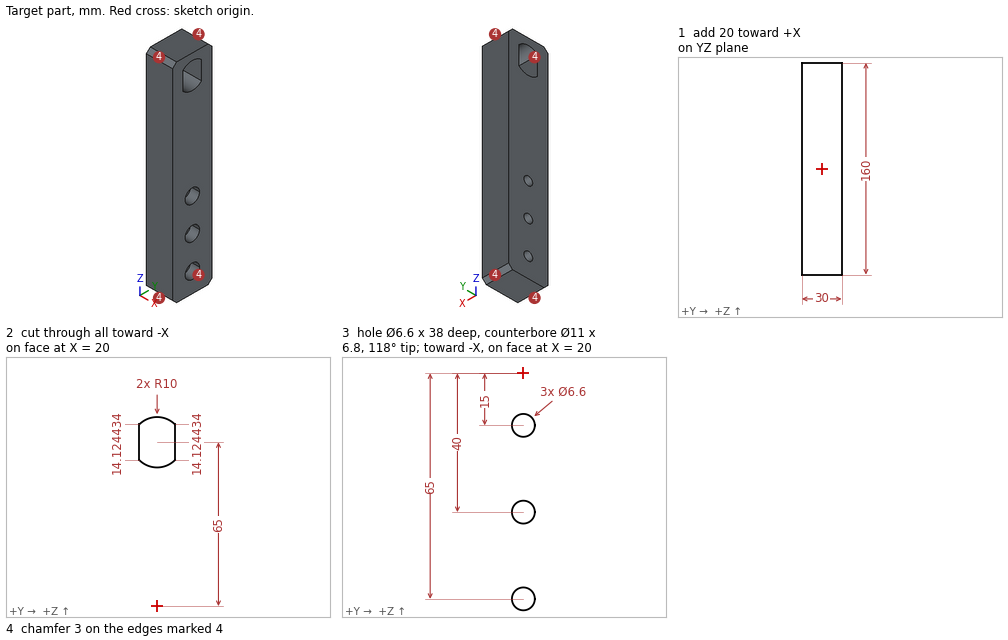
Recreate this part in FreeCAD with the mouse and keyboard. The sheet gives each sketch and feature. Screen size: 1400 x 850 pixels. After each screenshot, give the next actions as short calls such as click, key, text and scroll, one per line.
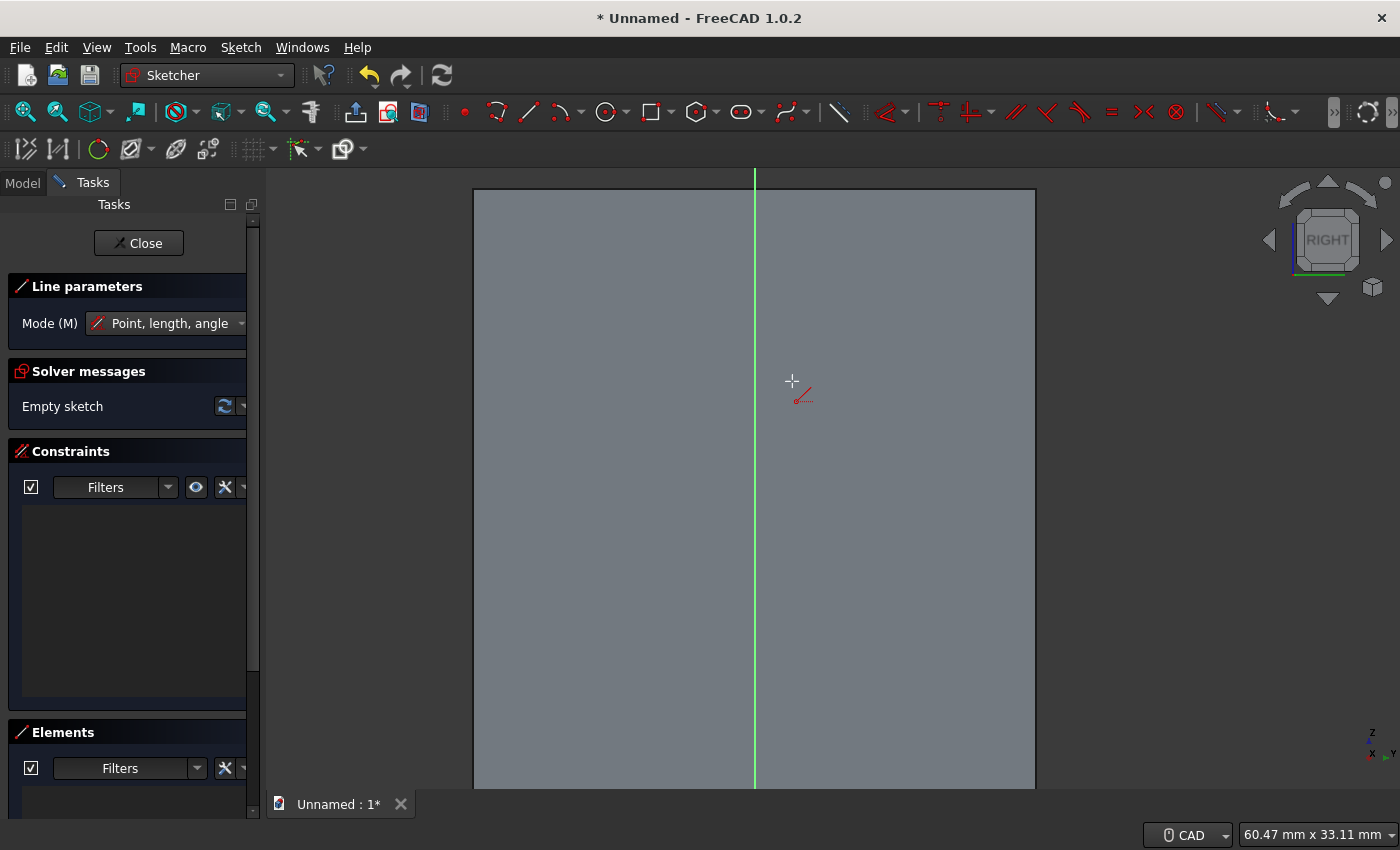
click(888, 603)
click(888, 338)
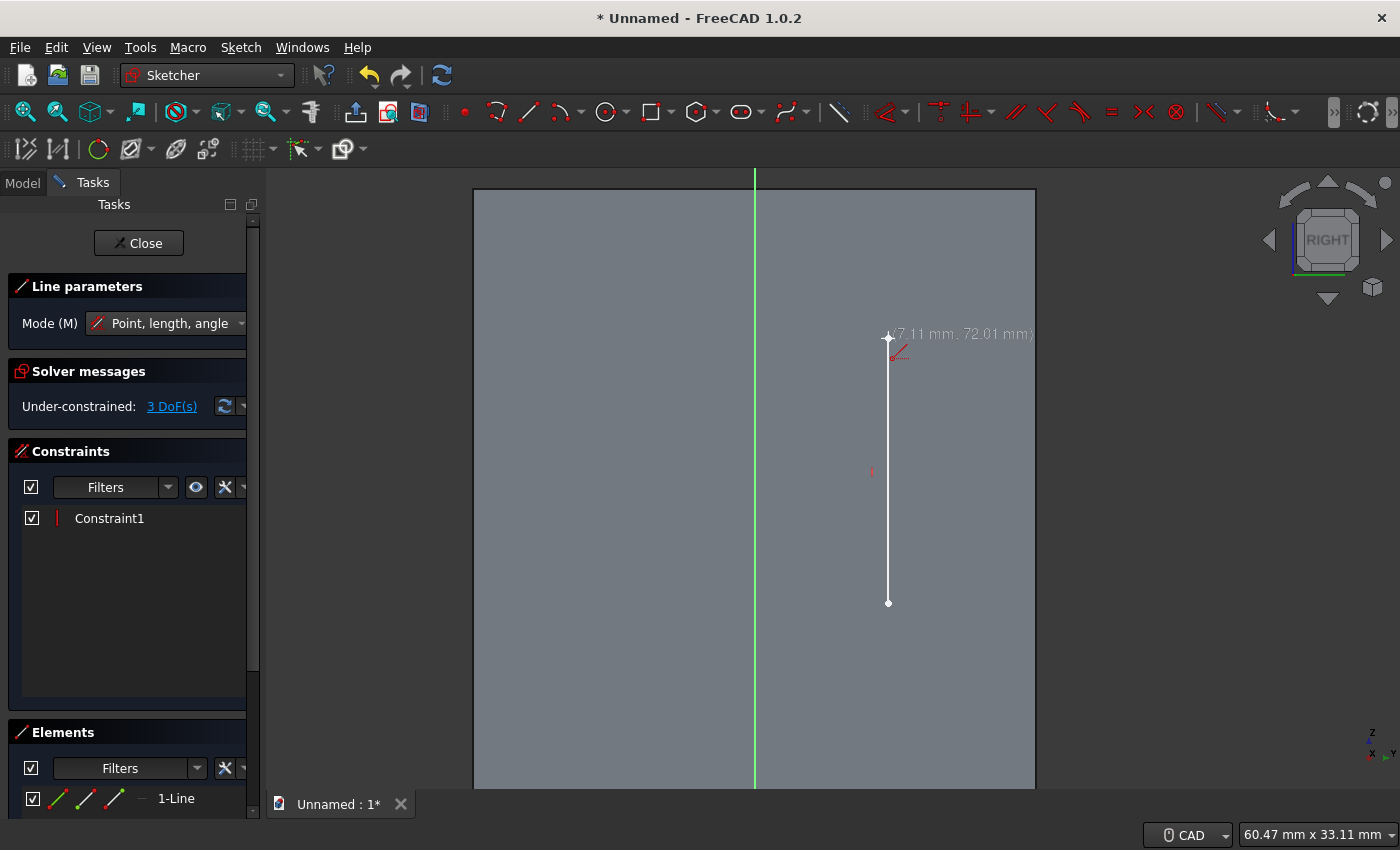
click(622, 338)
click(622, 603)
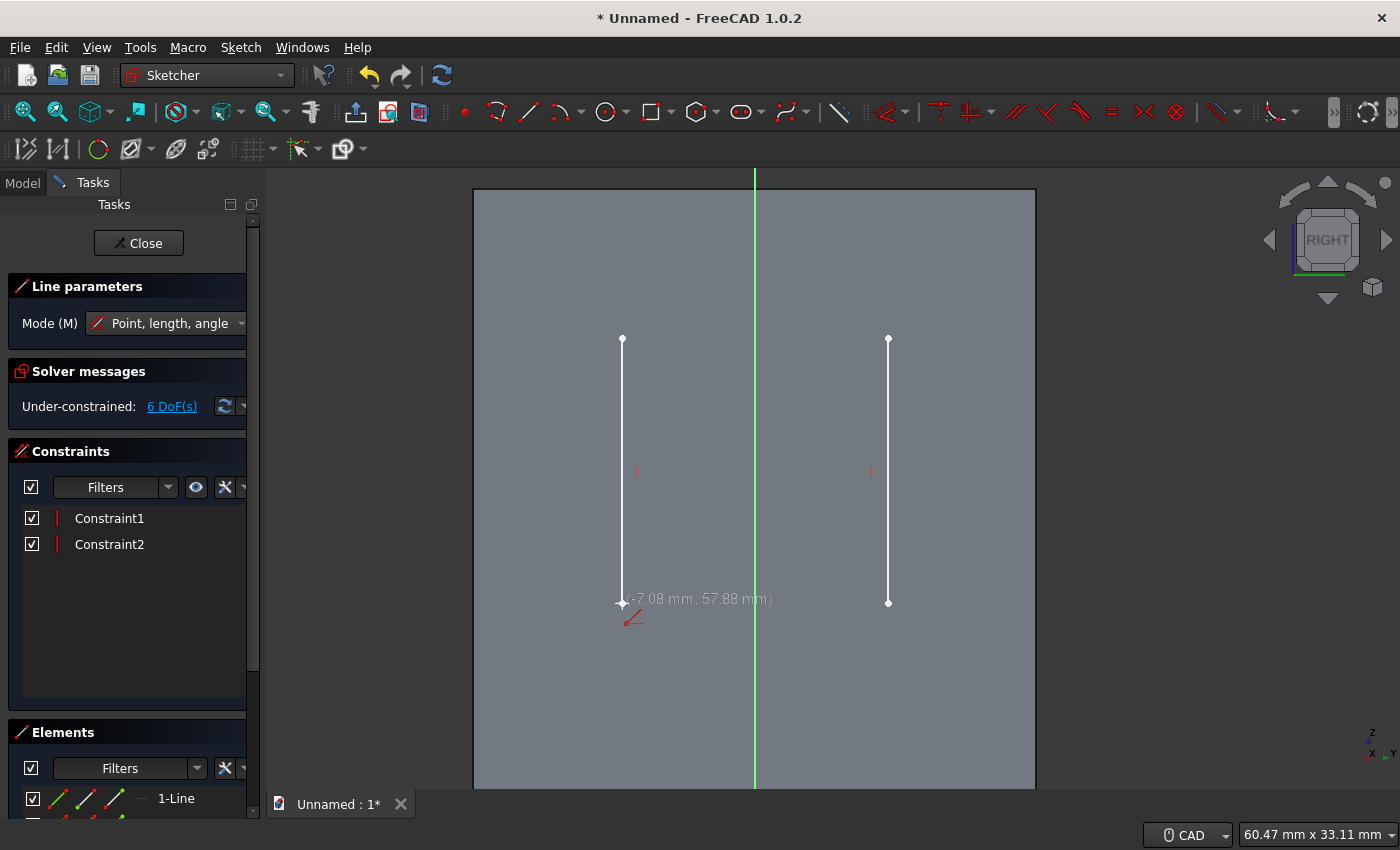
click(584, 112)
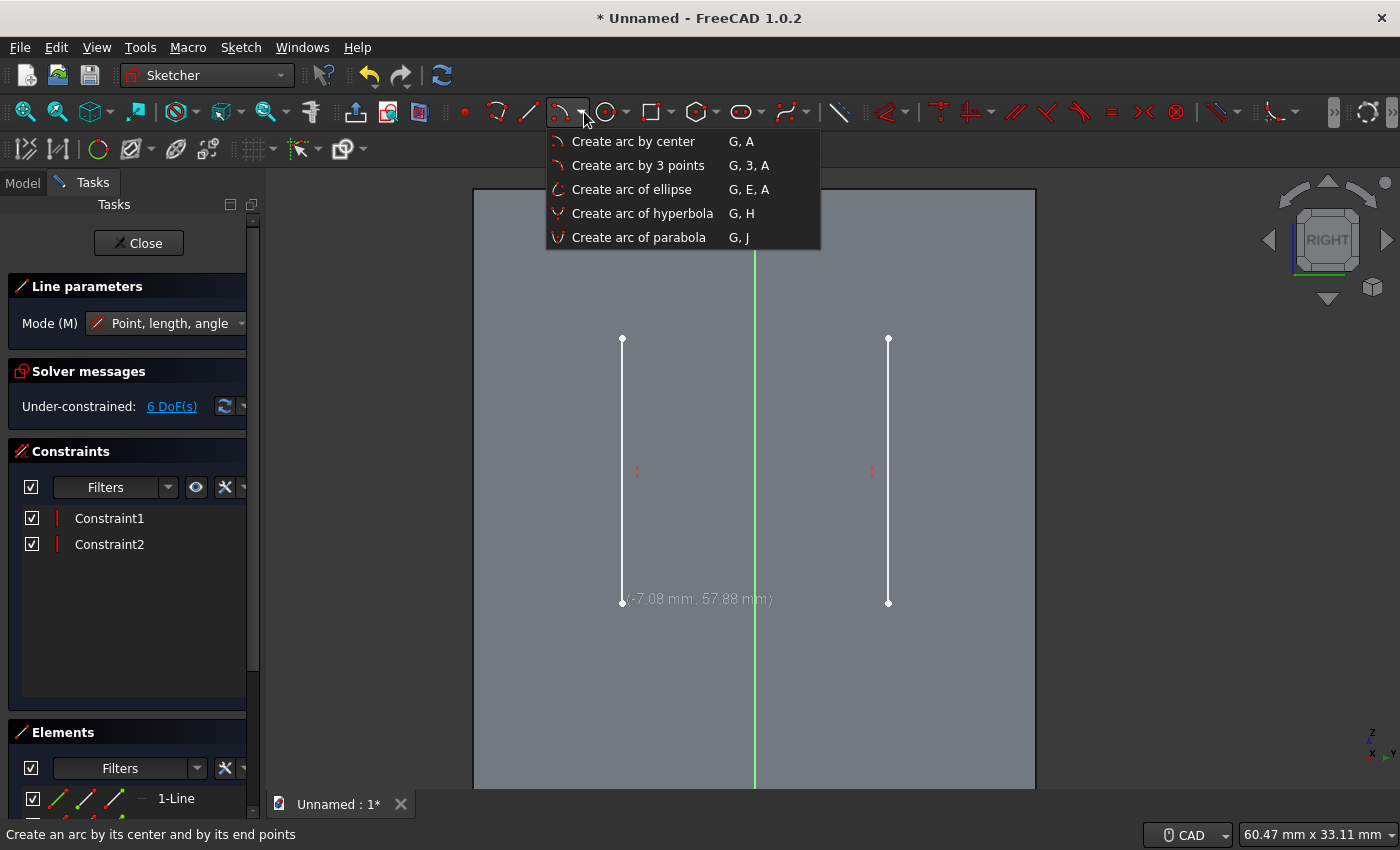
click(684, 165)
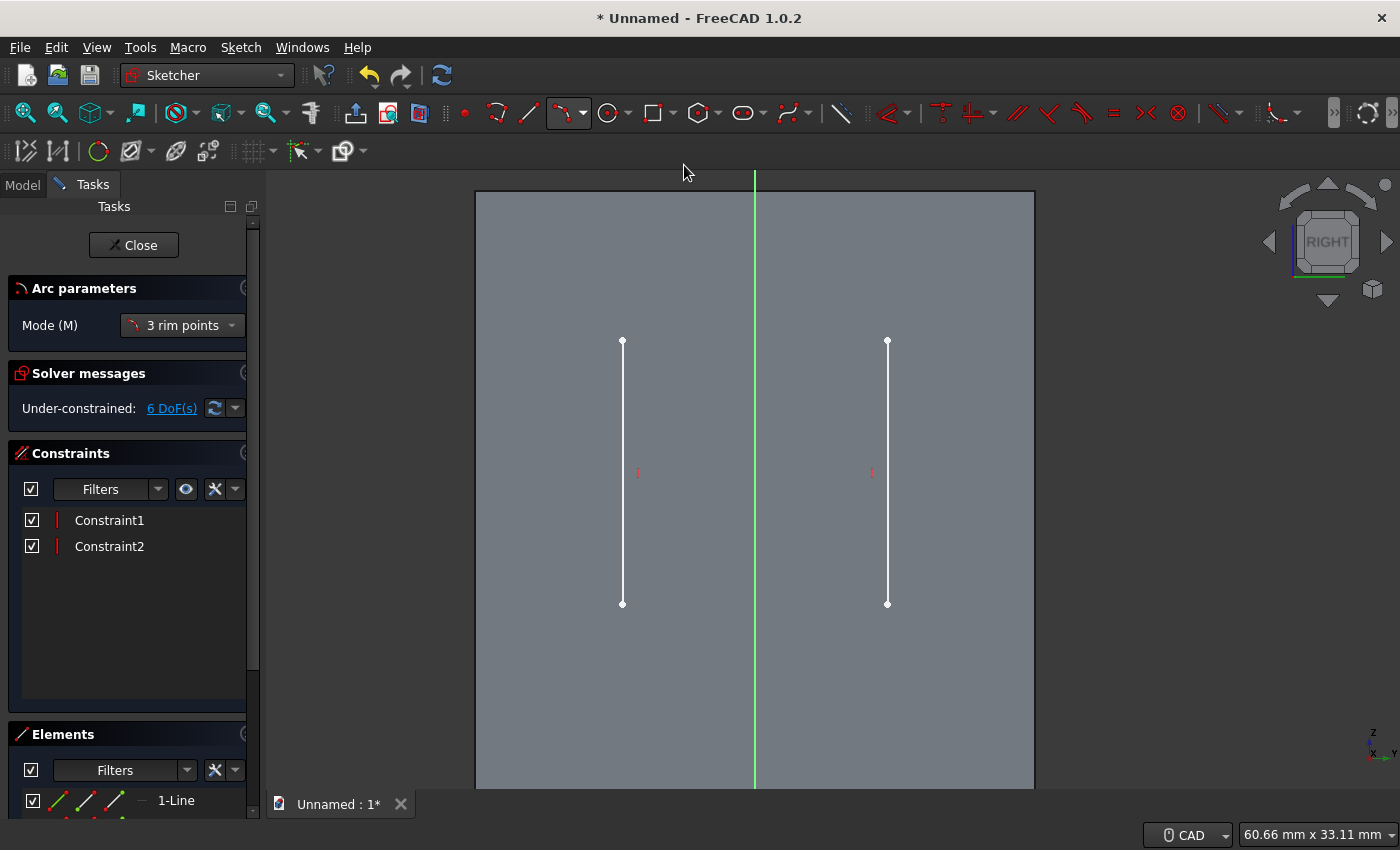
click(888, 340)
click(623, 340)
click(784, 287)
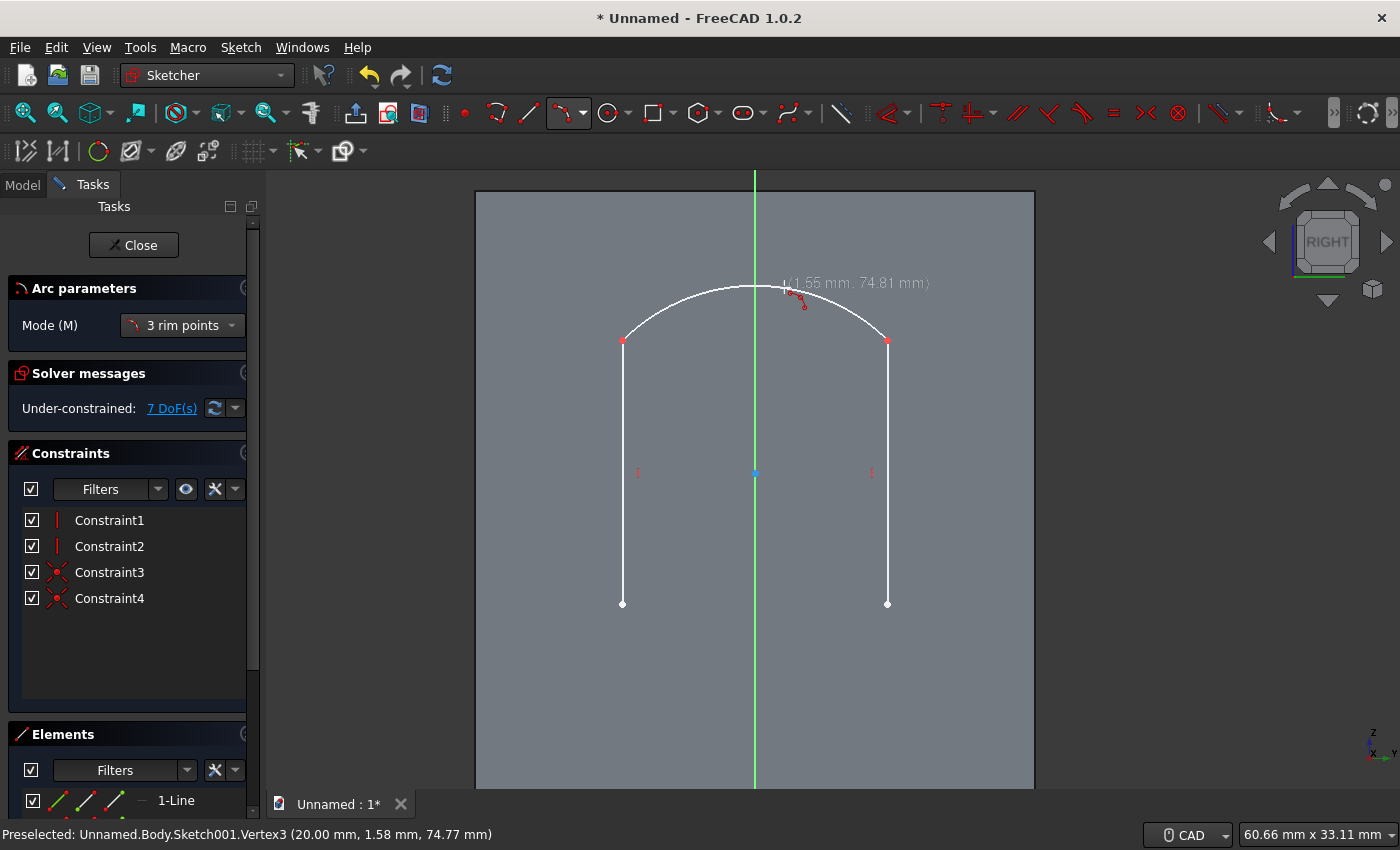
click(623, 605)
click(888, 605)
click(726, 656)
key(Escape)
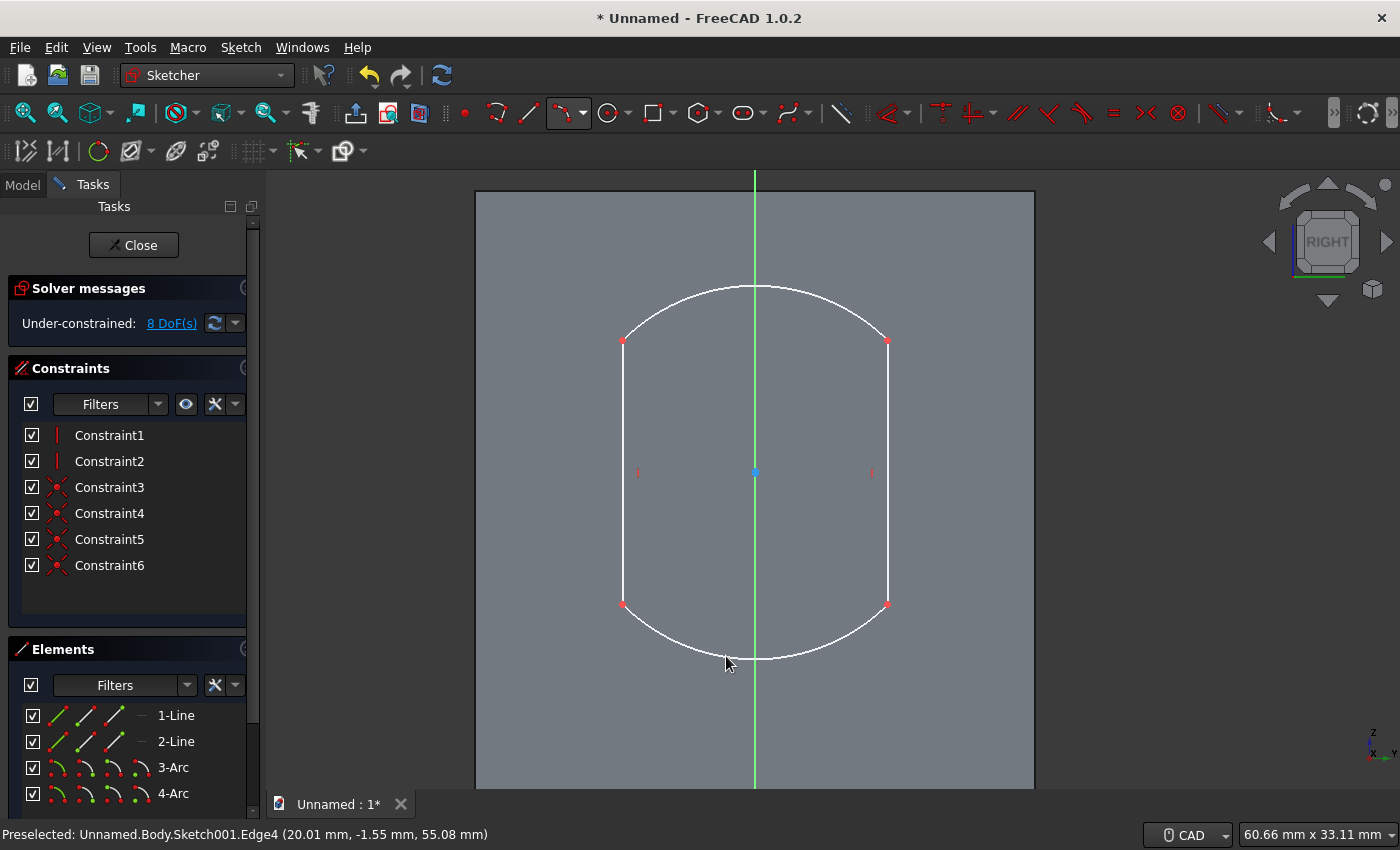
click(813, 295)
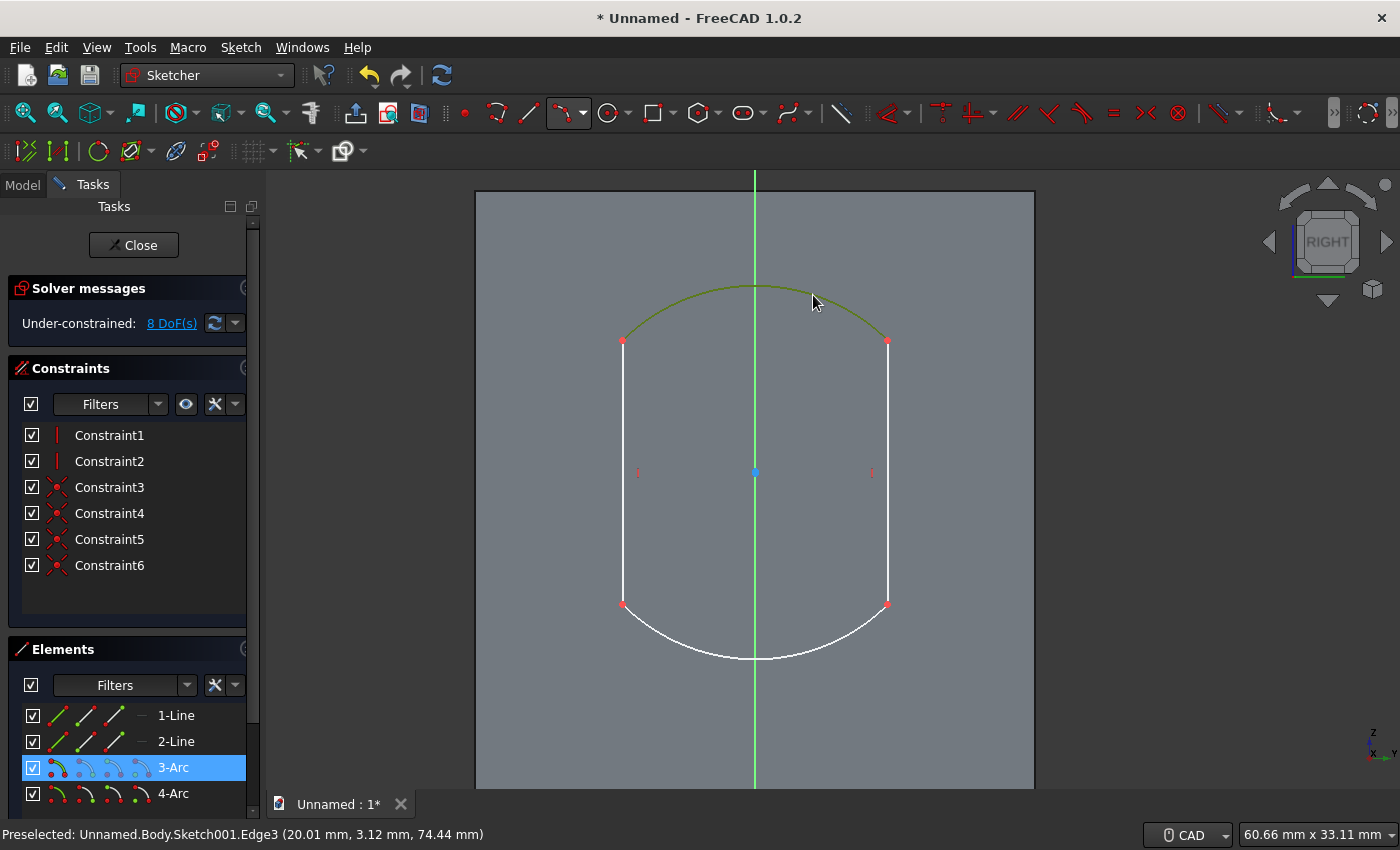
click(697, 650)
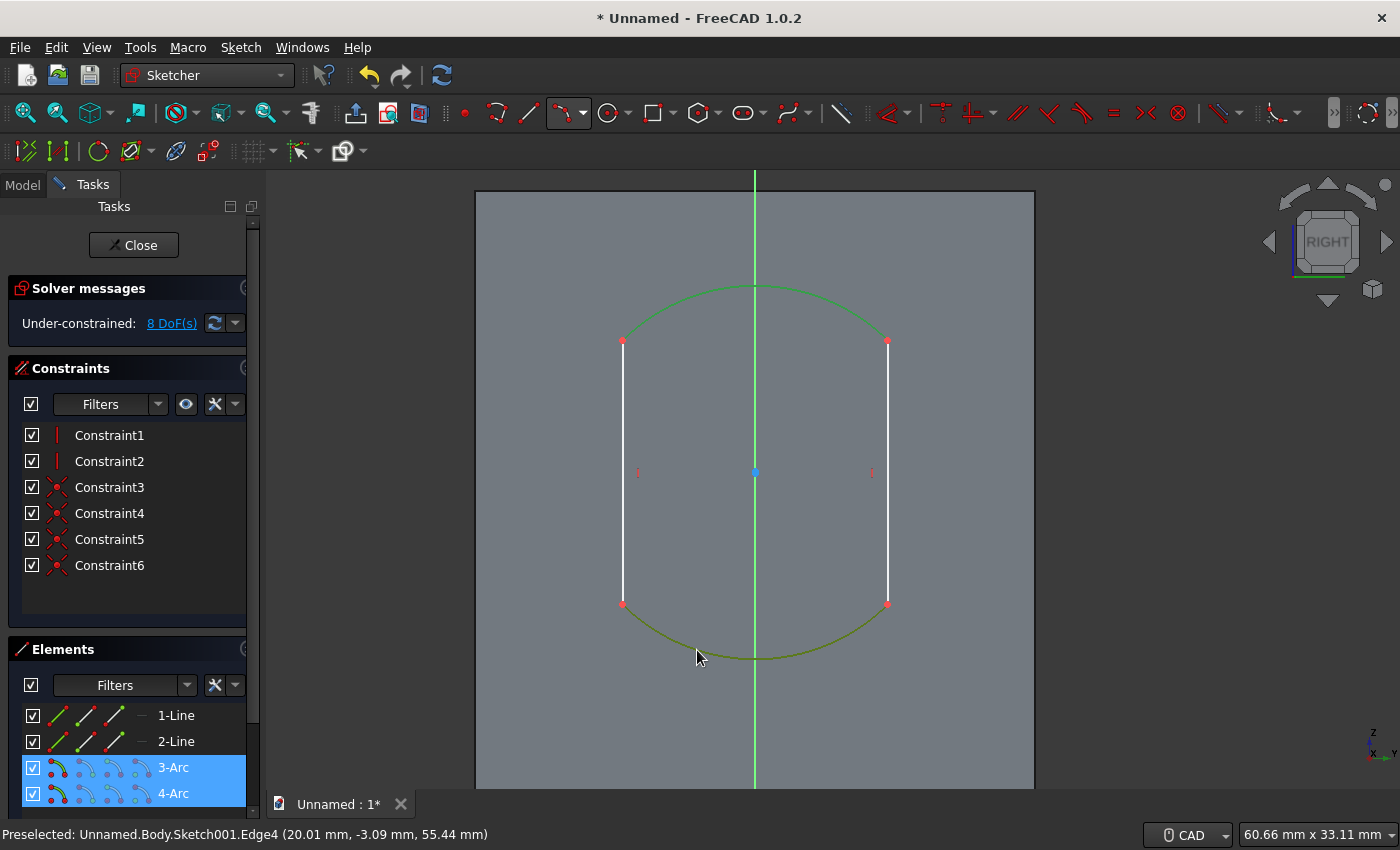
key(c)